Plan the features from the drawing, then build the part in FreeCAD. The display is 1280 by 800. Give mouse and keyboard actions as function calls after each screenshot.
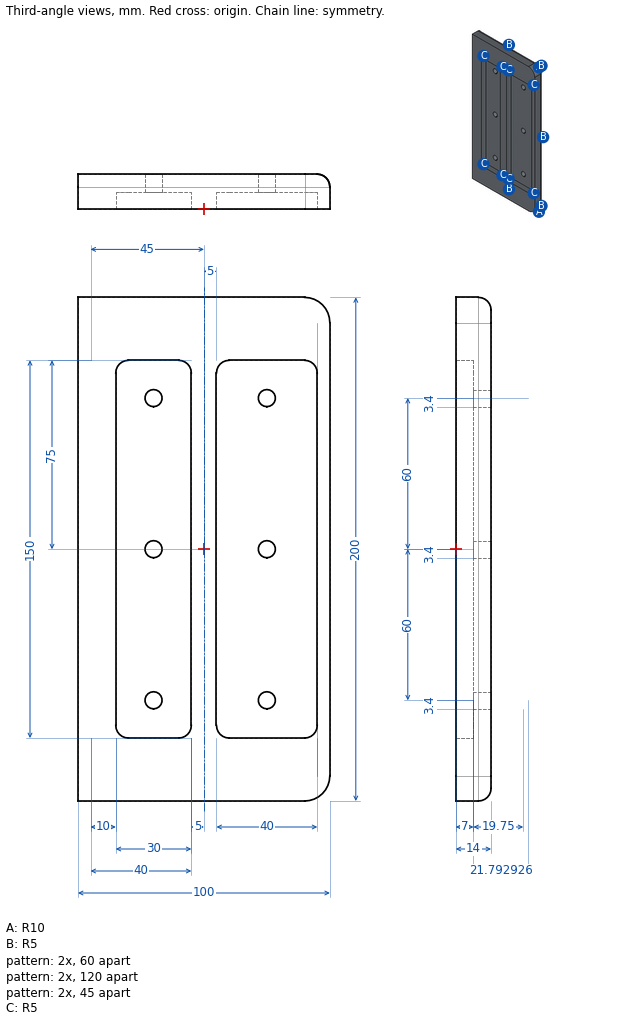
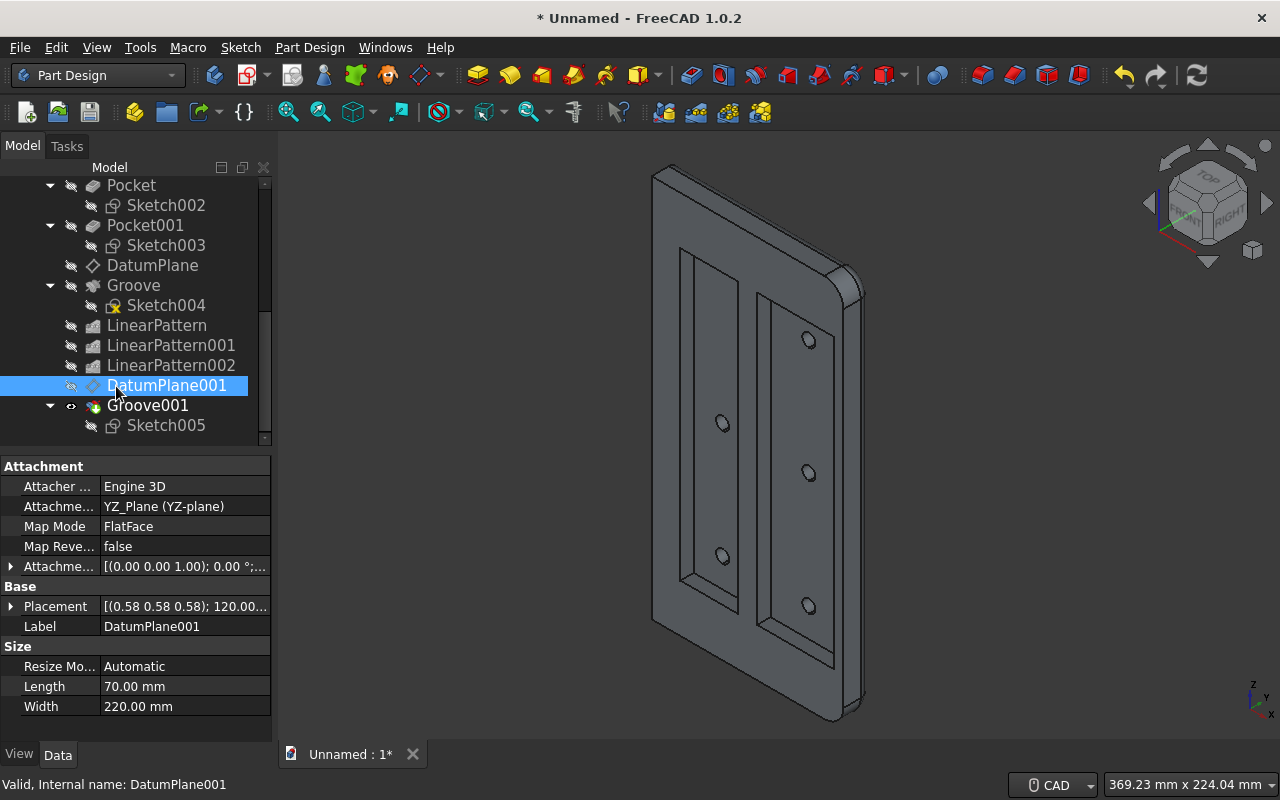
scroll(140, 301, down, 3)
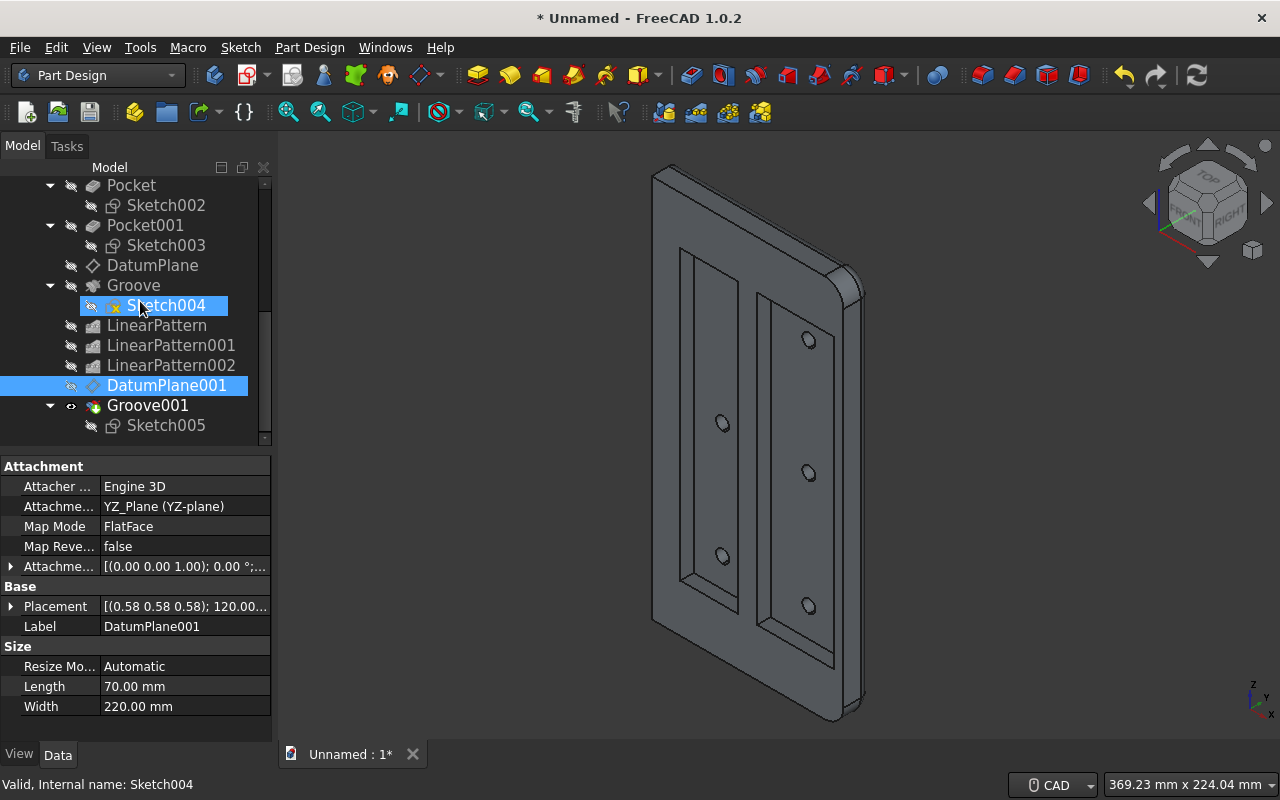
scroll(140, 301, up, 15)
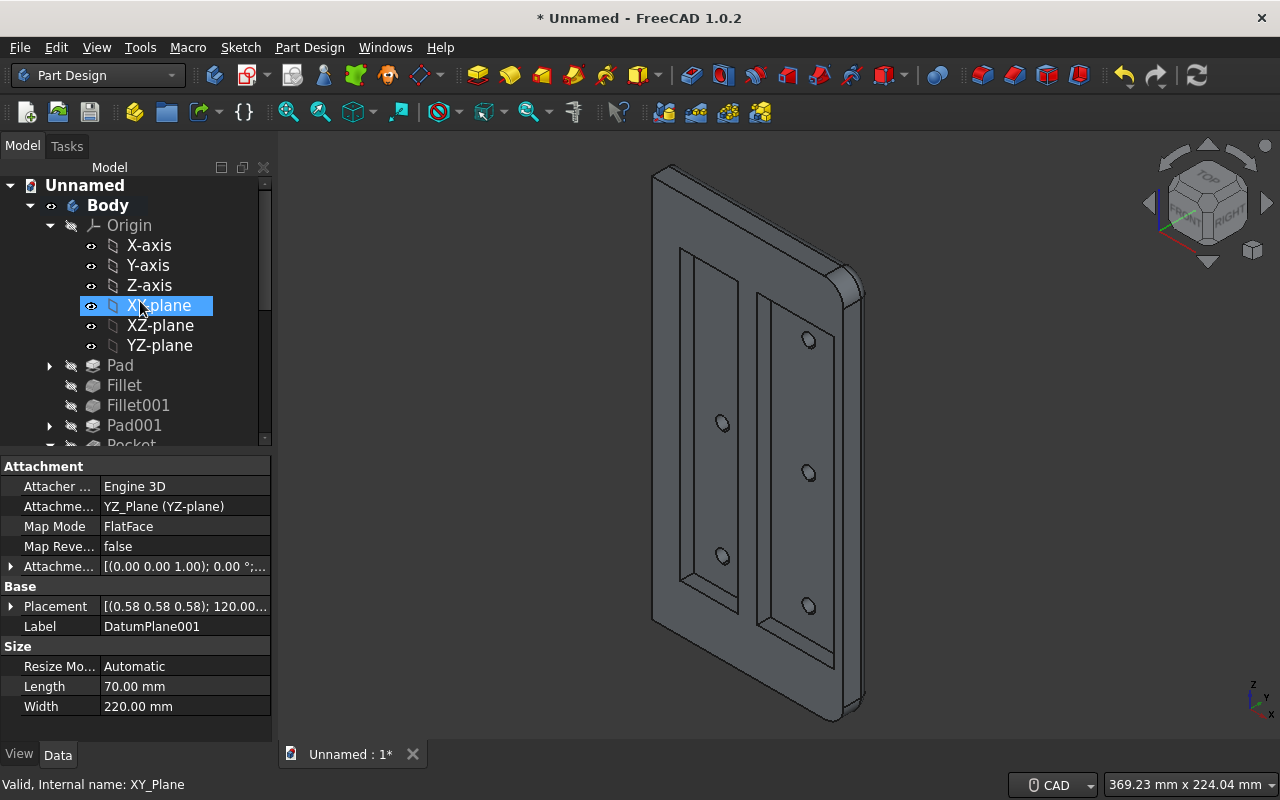
click(136, 346)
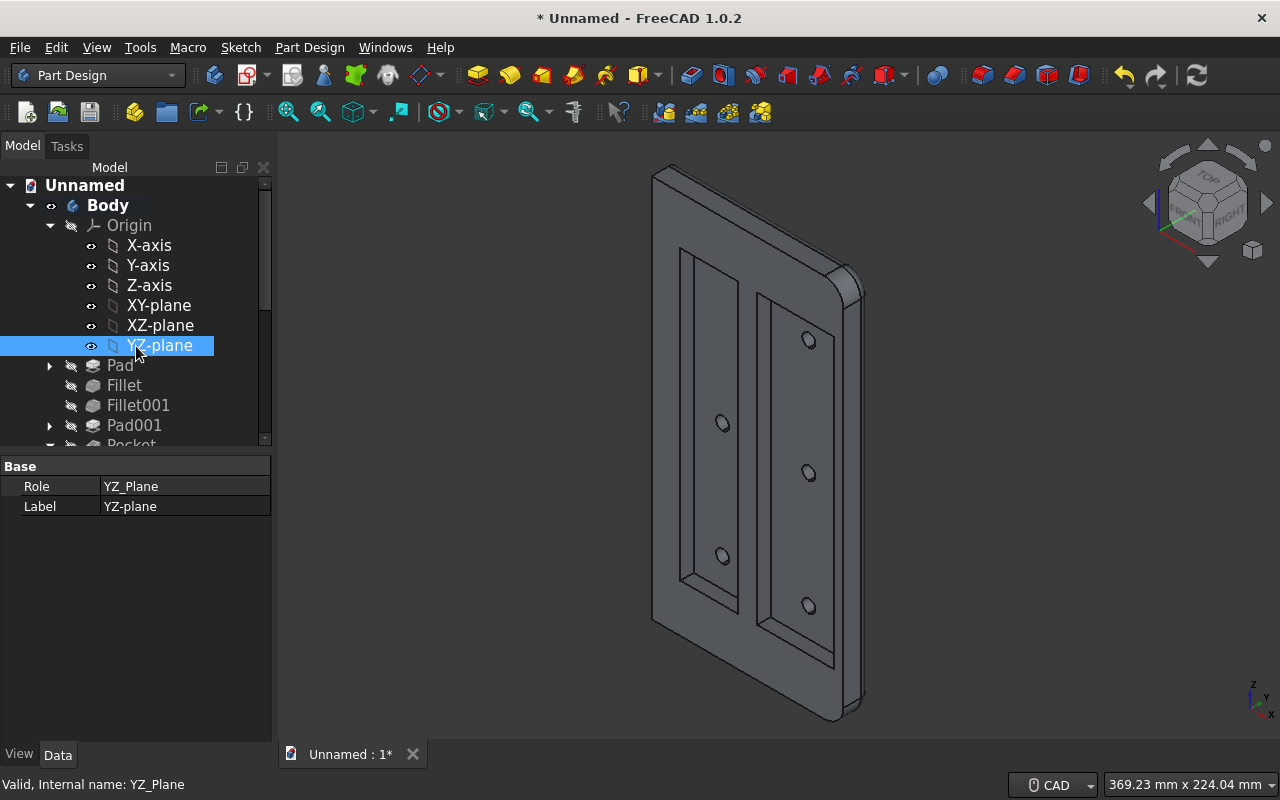
click(420, 76)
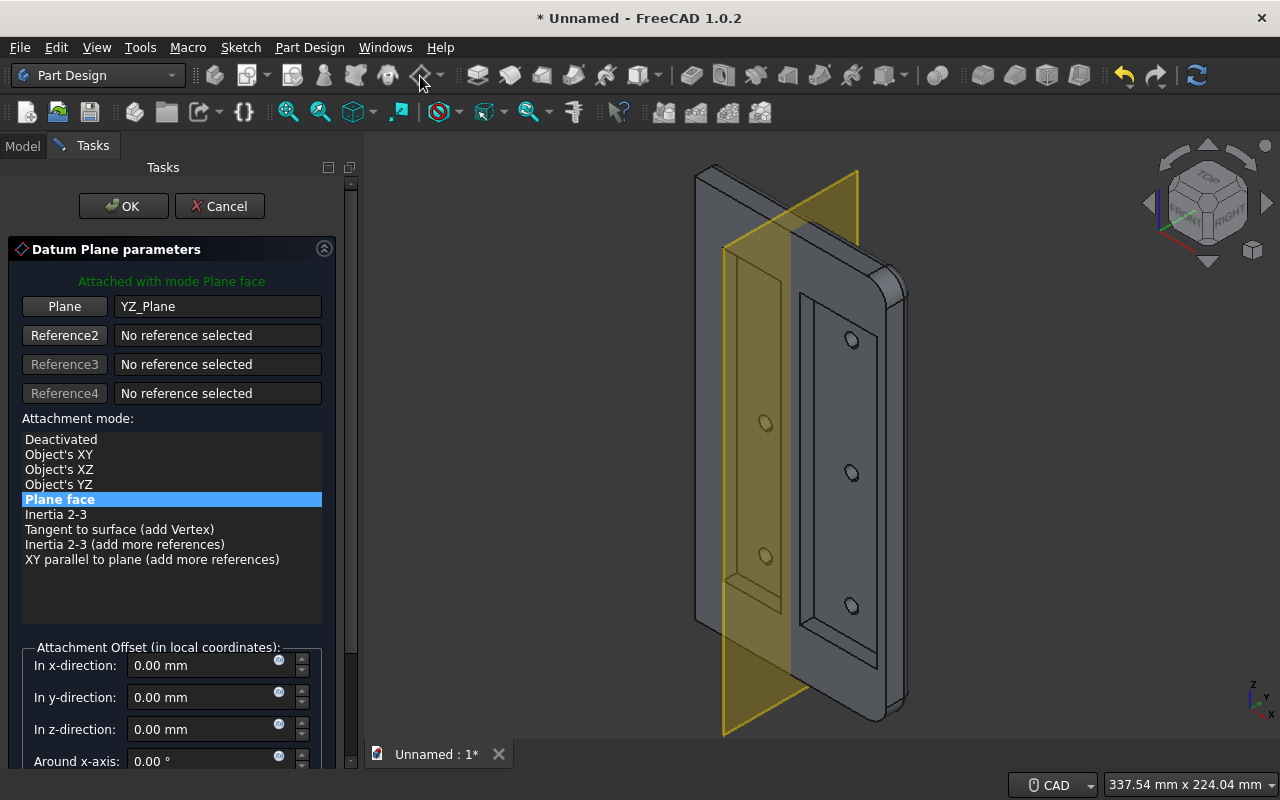
triple_click(210, 729)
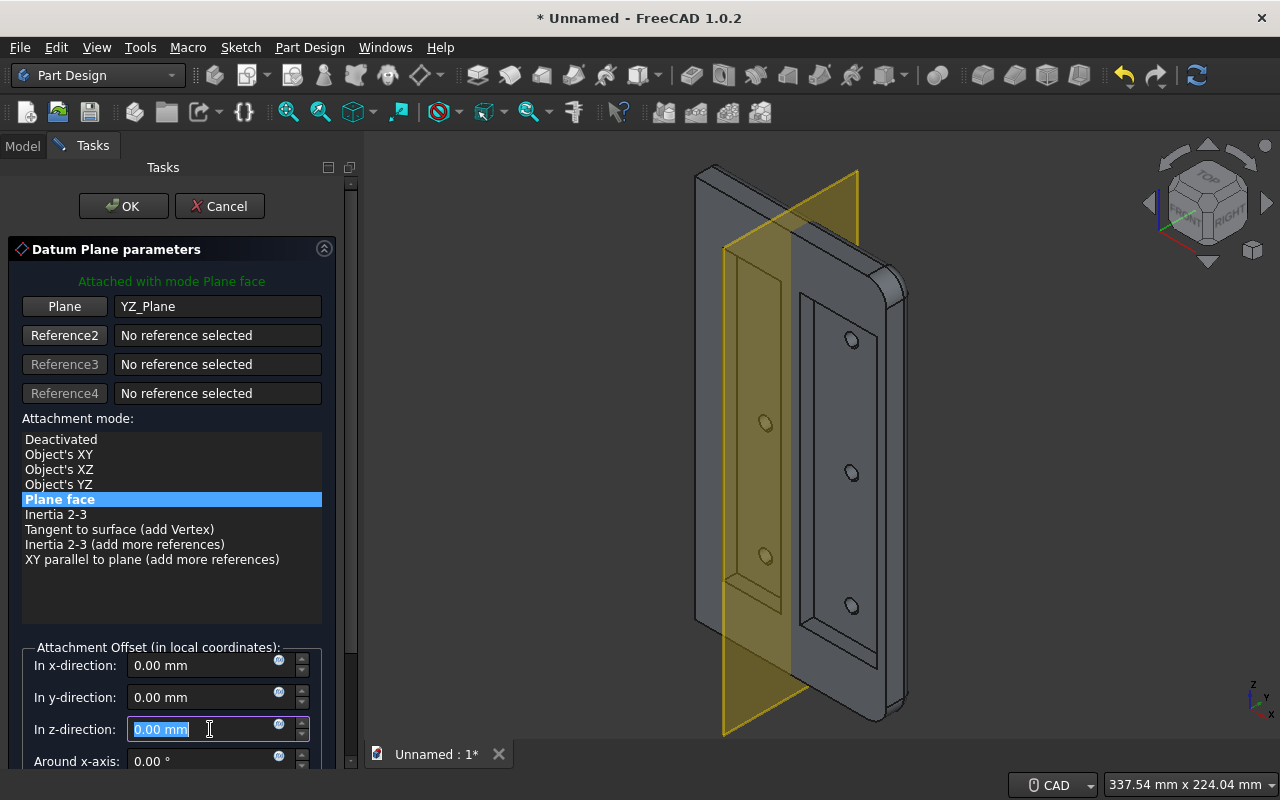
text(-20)
key(Tab)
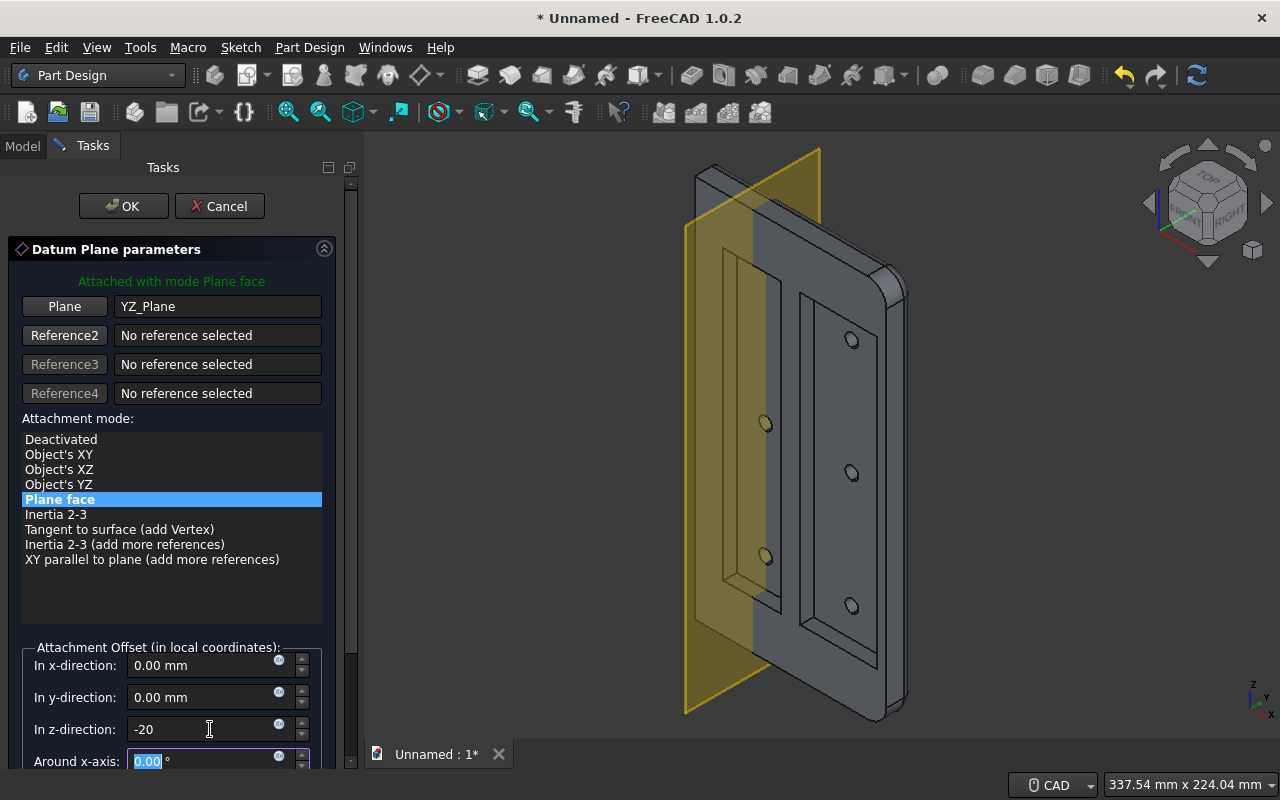
click(124, 206)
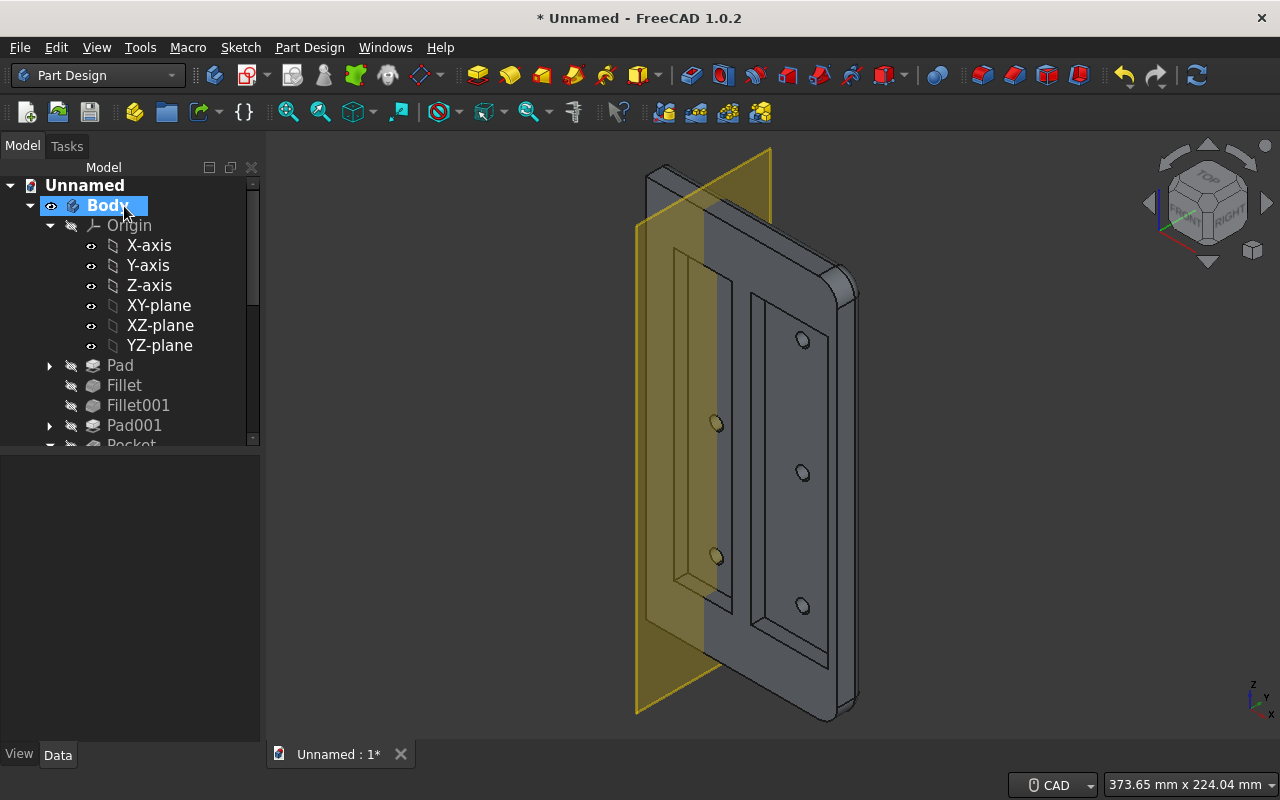
scroll(100, 321, down, 3)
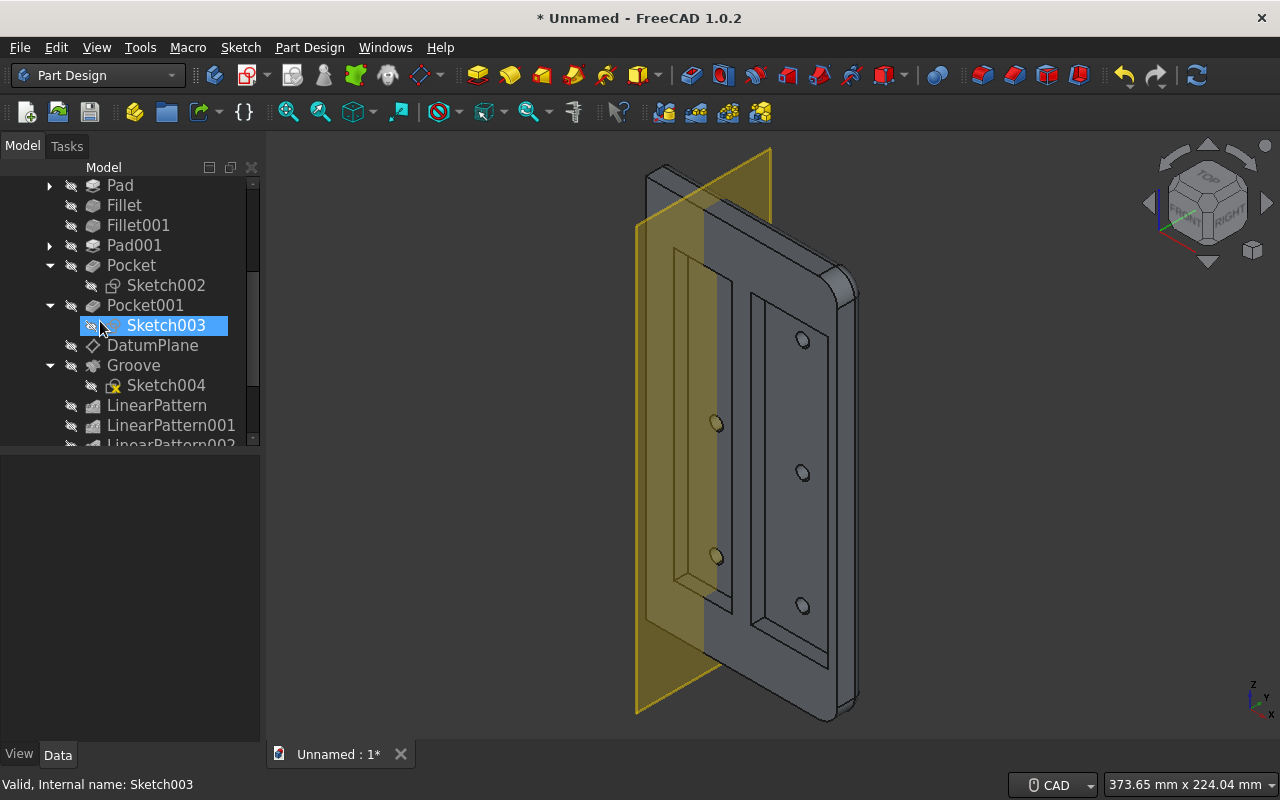
scroll(140, 321, up, 15)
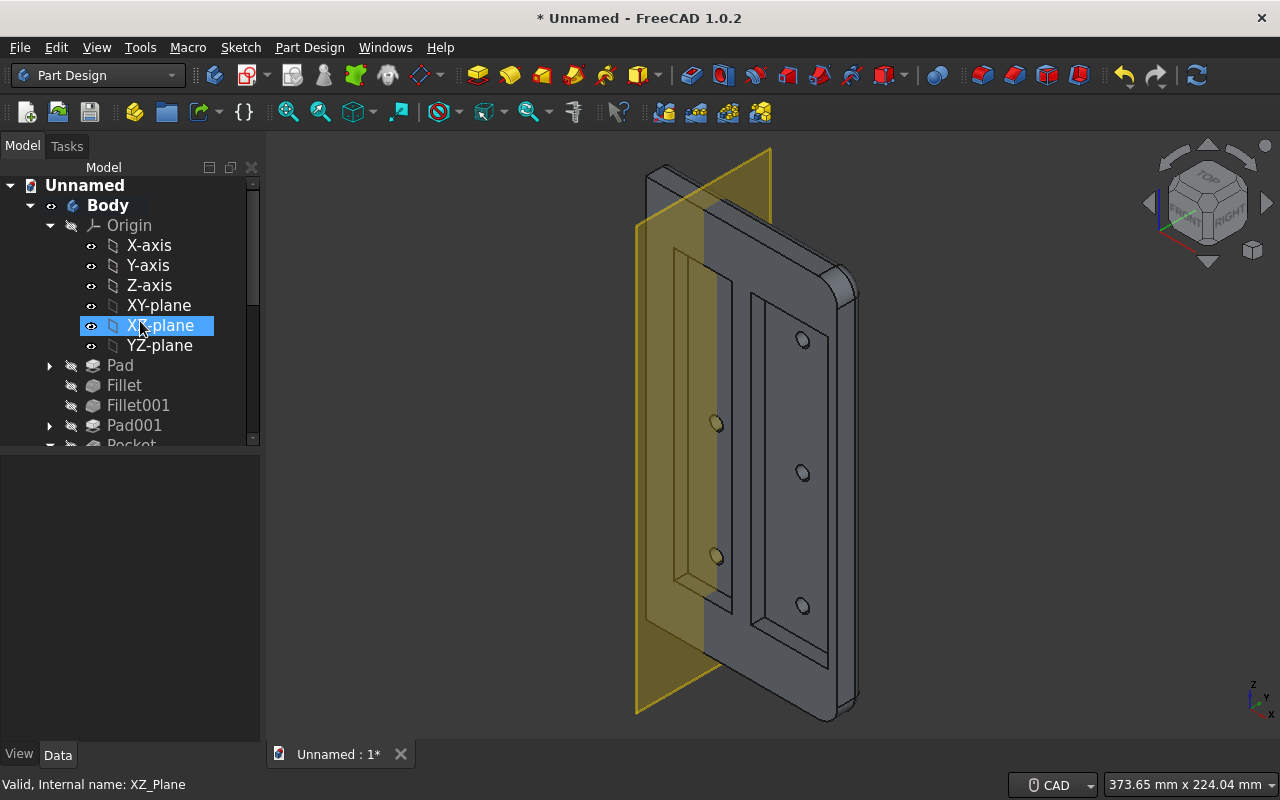
scroll(100, 321, down, 6)